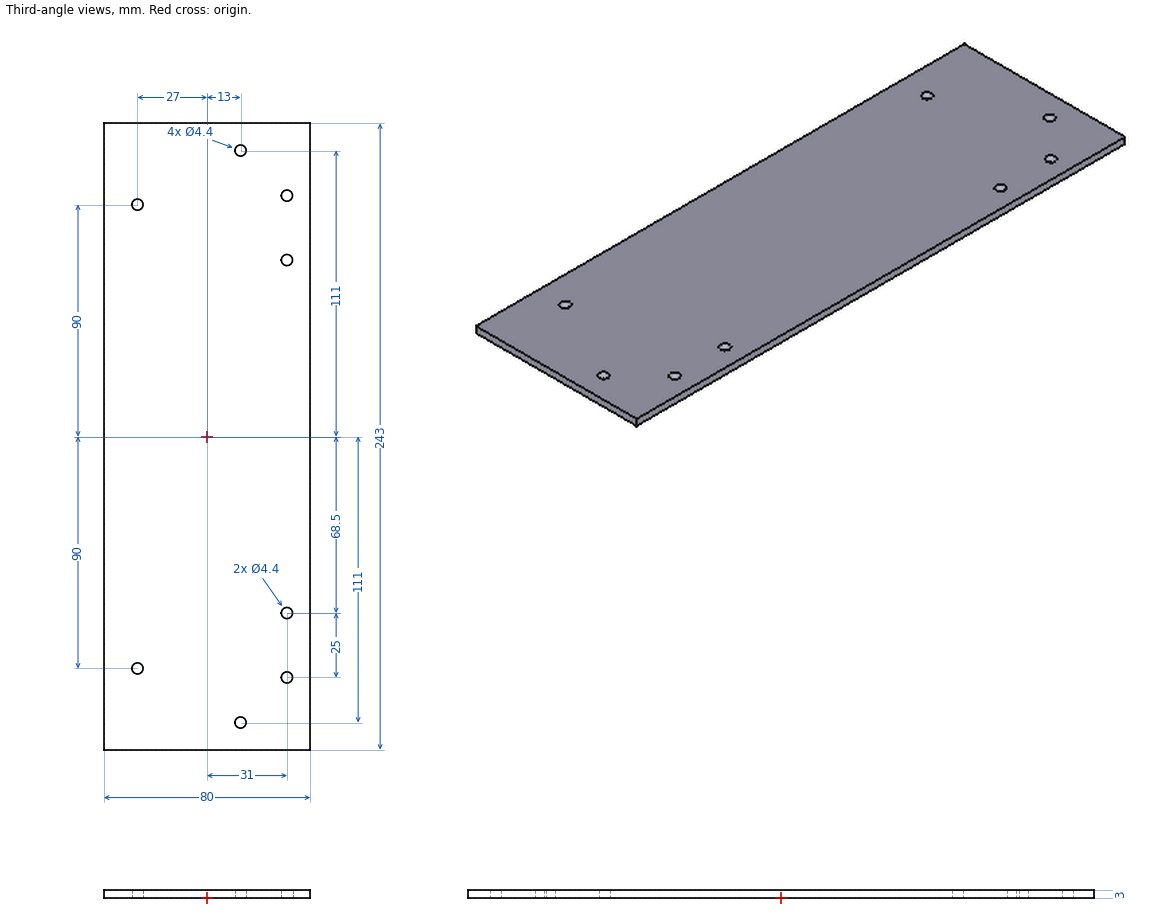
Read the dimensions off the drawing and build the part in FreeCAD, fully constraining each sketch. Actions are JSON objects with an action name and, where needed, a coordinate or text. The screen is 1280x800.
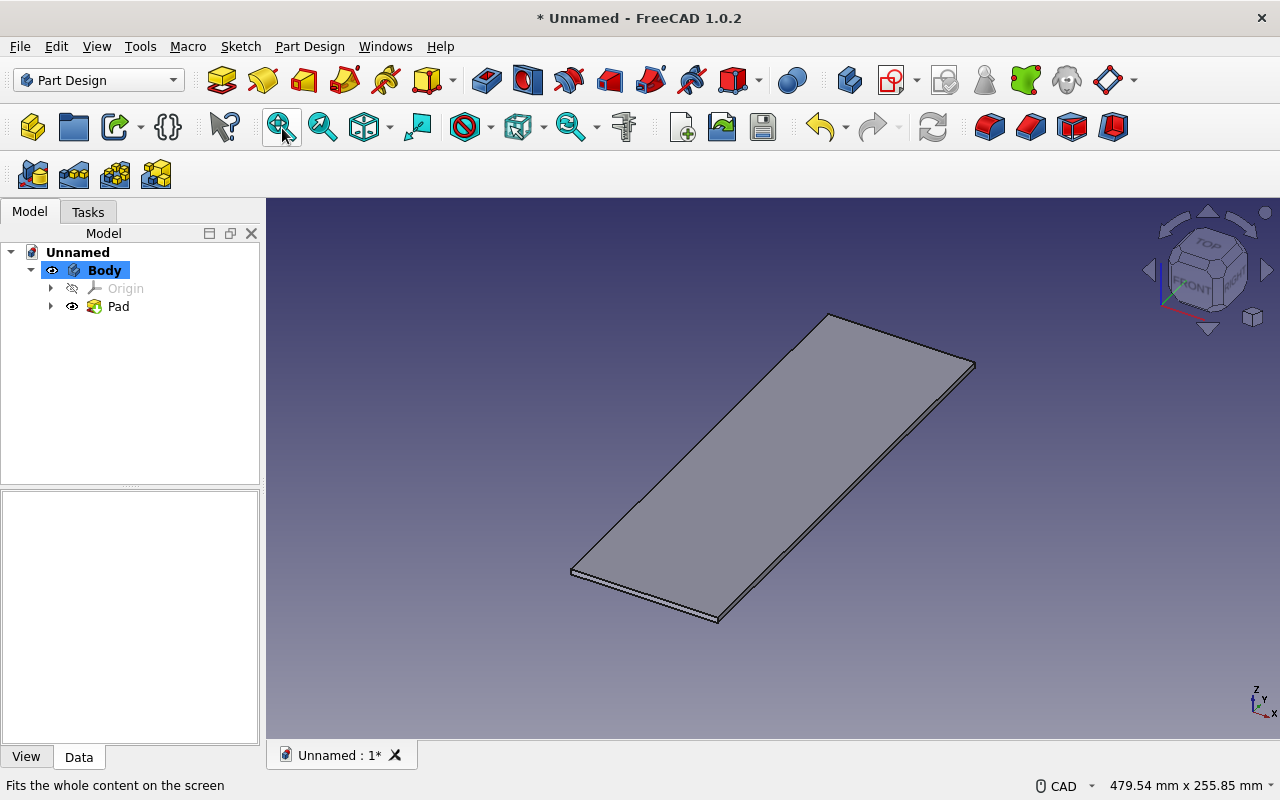
{"action": "key", "text": "5"}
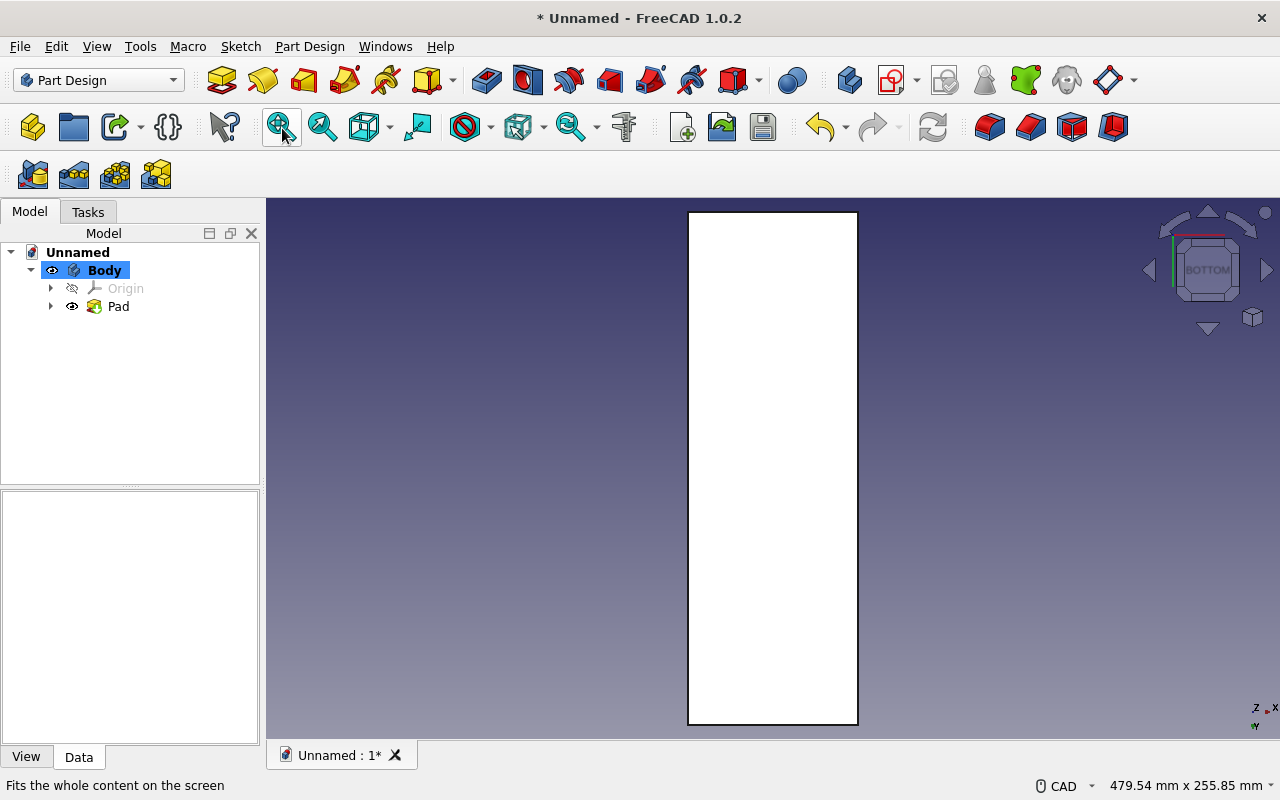
{"action": "left_click", "coordinate": [773, 614]}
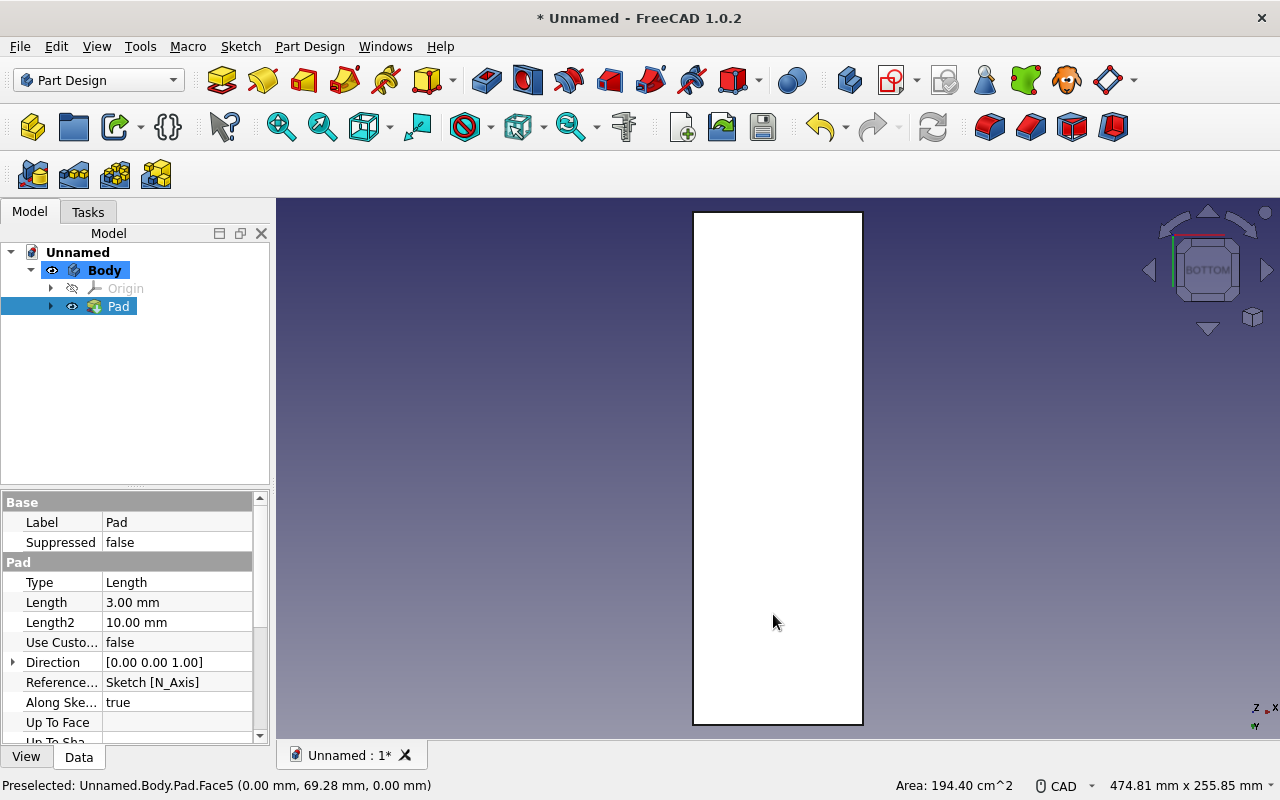
{"action": "left_click", "coordinate": [890, 80]}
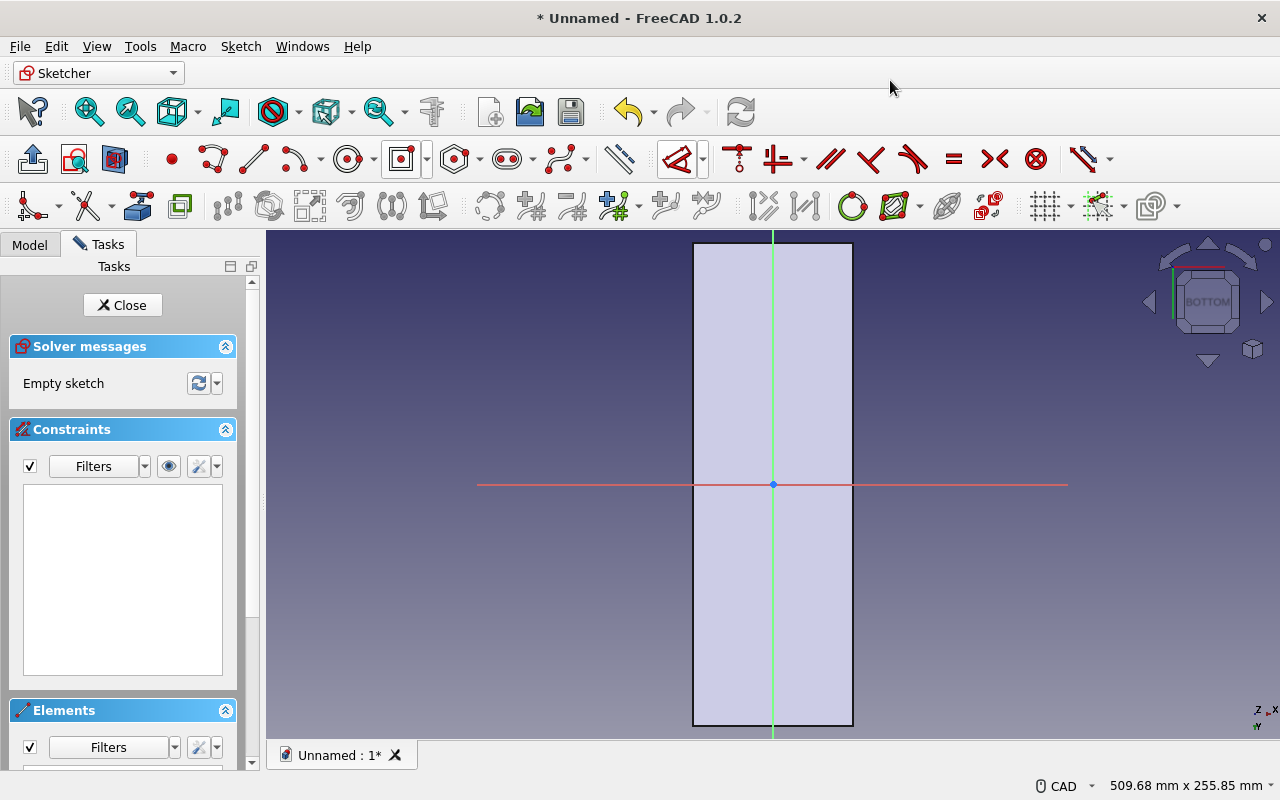
{"action": "scroll", "coordinate": [868, 283], "scroll_direction": "up", "scroll_amount": 8}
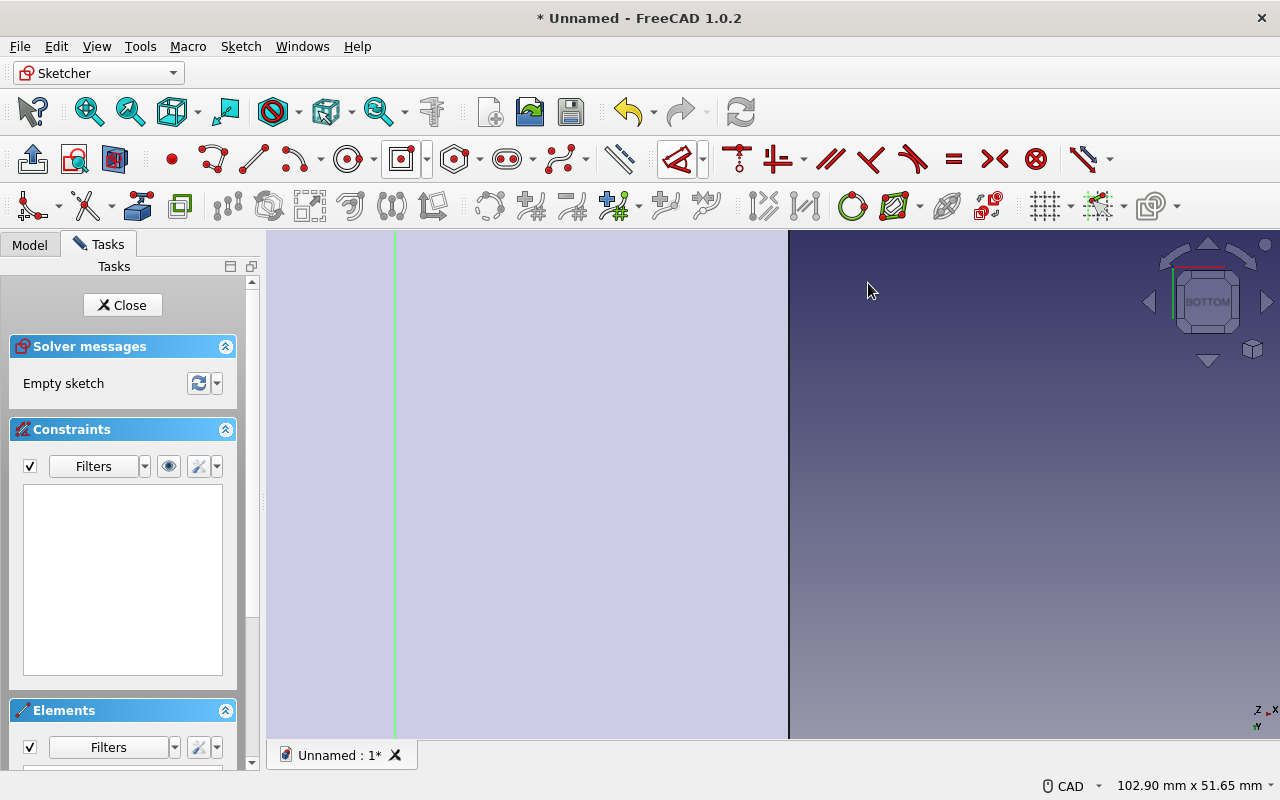
{"action": "left_click", "coordinate": [348, 160]}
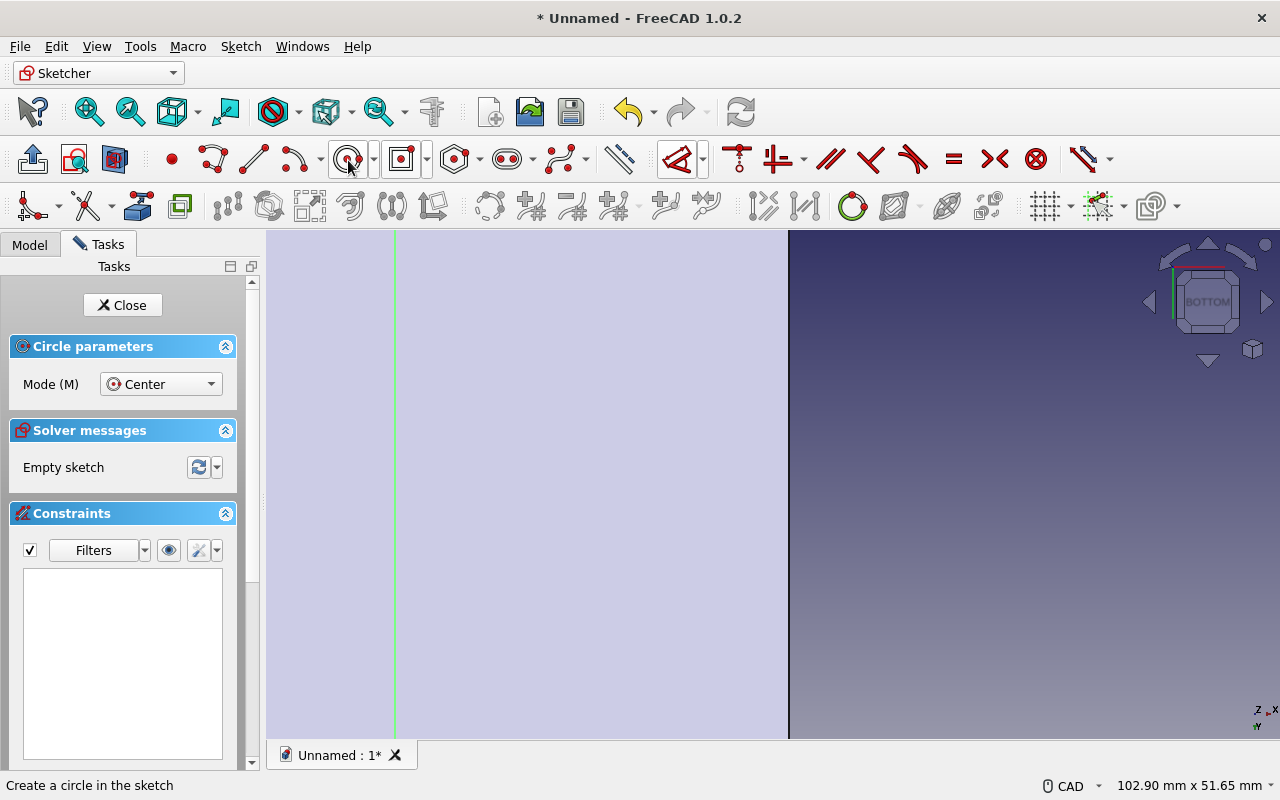
{"action": "left_click", "coordinate": [701, 606]}
{"action": "left_click", "coordinate": [716, 590]}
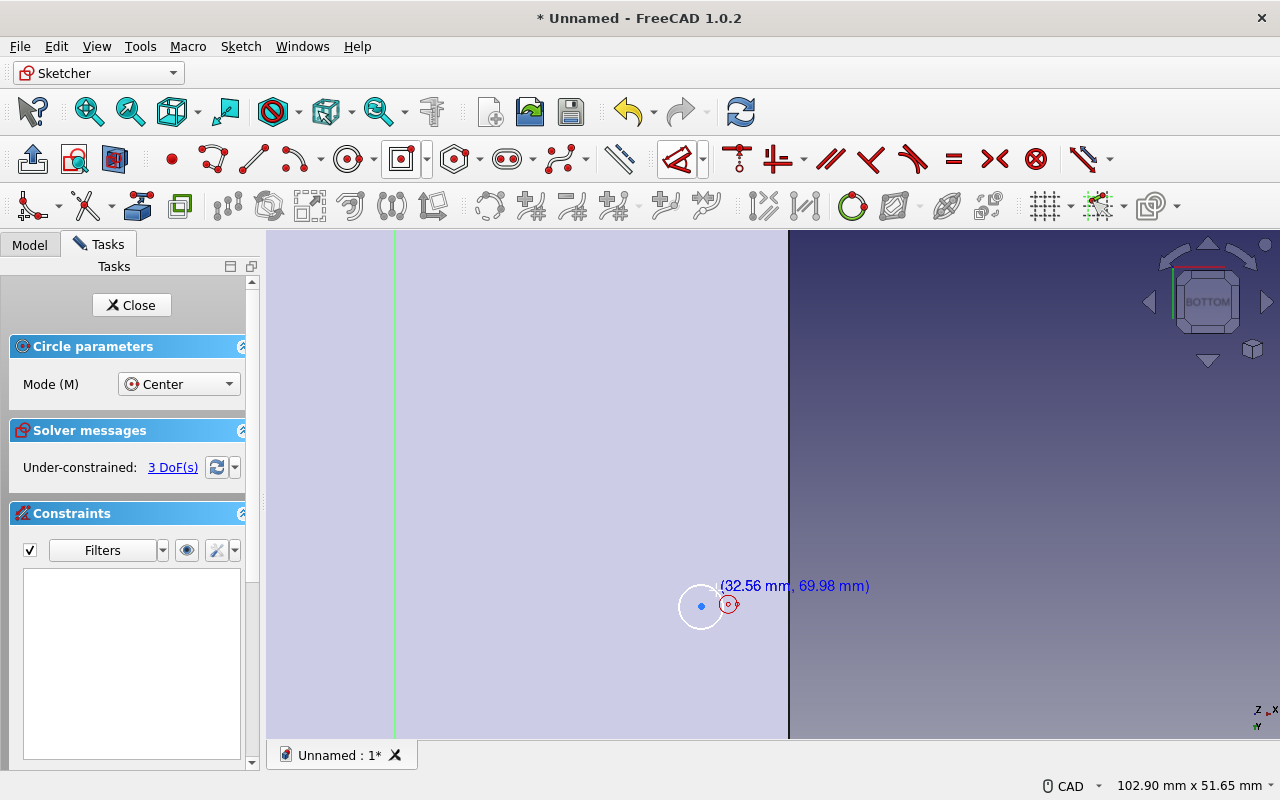
{"action": "left_click", "coordinate": [701, 359]}
{"action": "left_click", "coordinate": [716, 344]}
{"action": "key", "text": "Escape"}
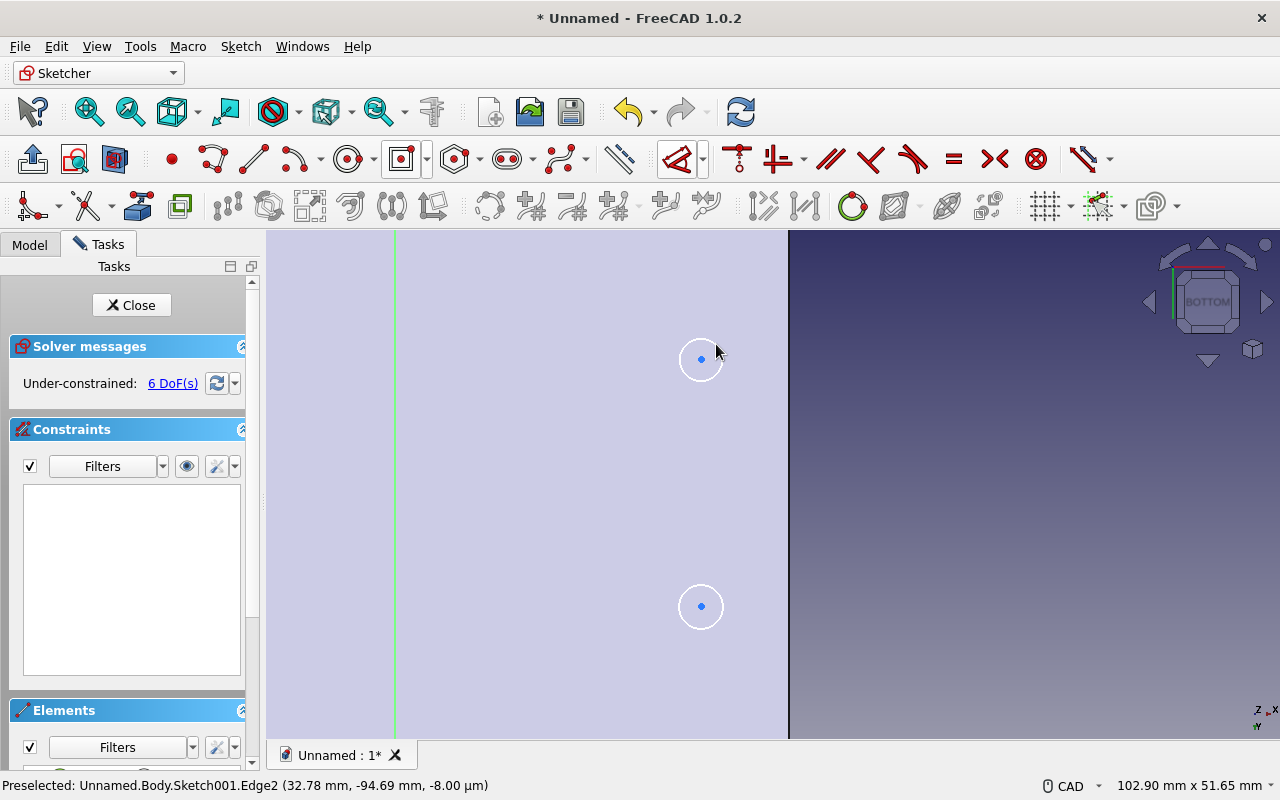
{"action": "left_click", "coordinate": [716, 591]}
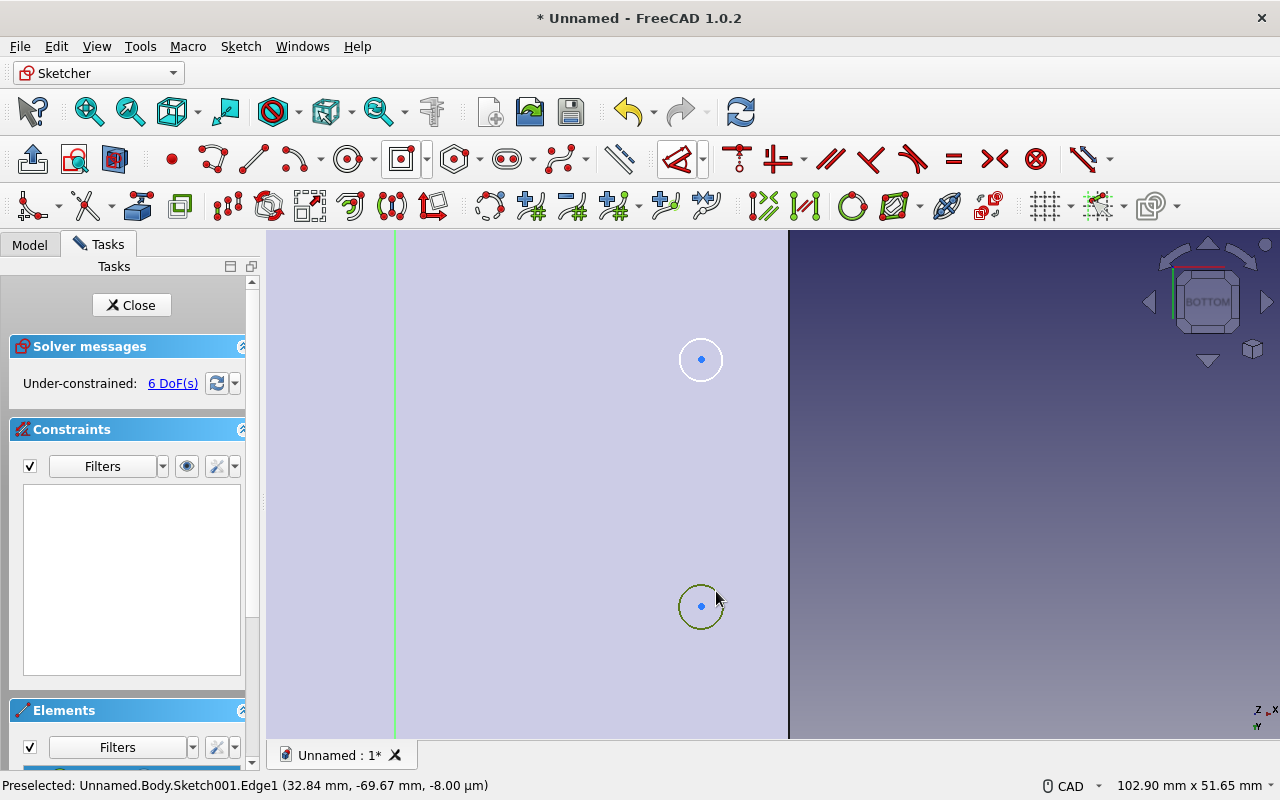
{"action": "left_click", "coordinate": [716, 345]}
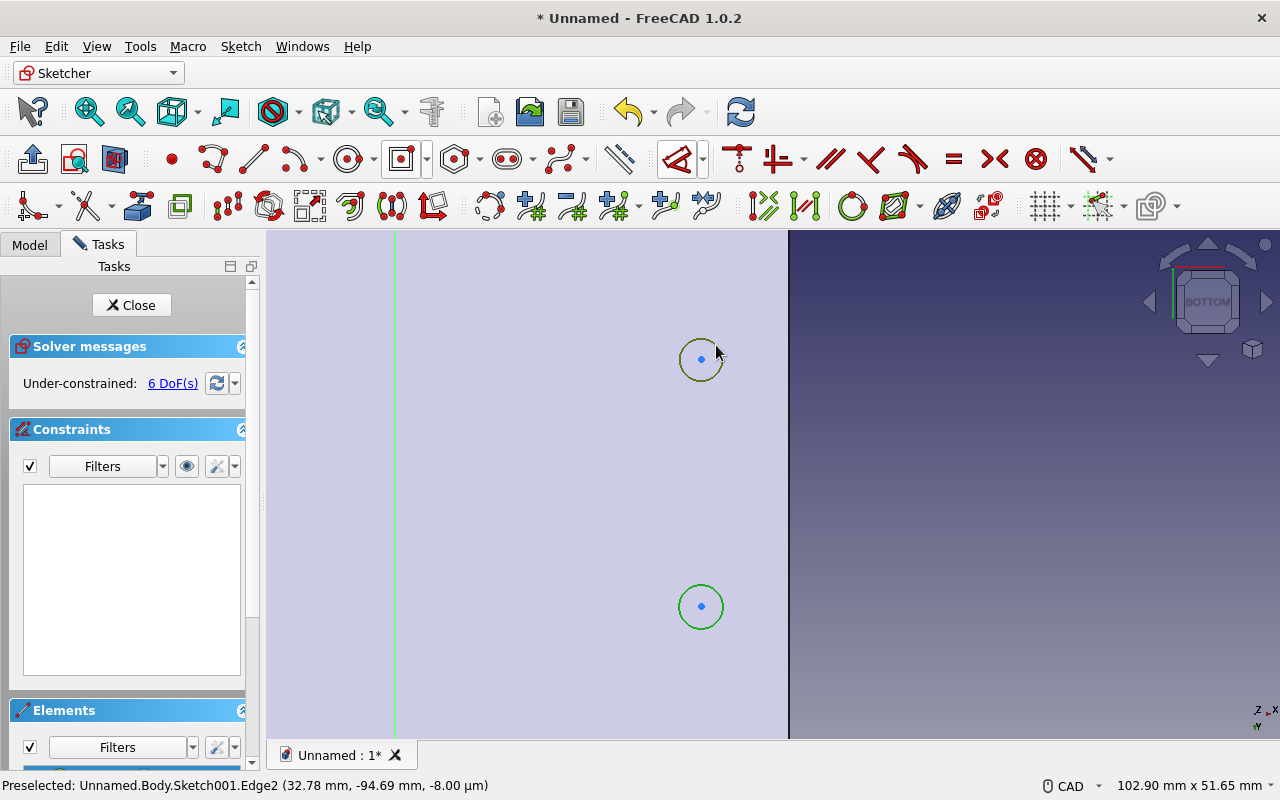
{"action": "left_click", "coordinate": [954, 160]}